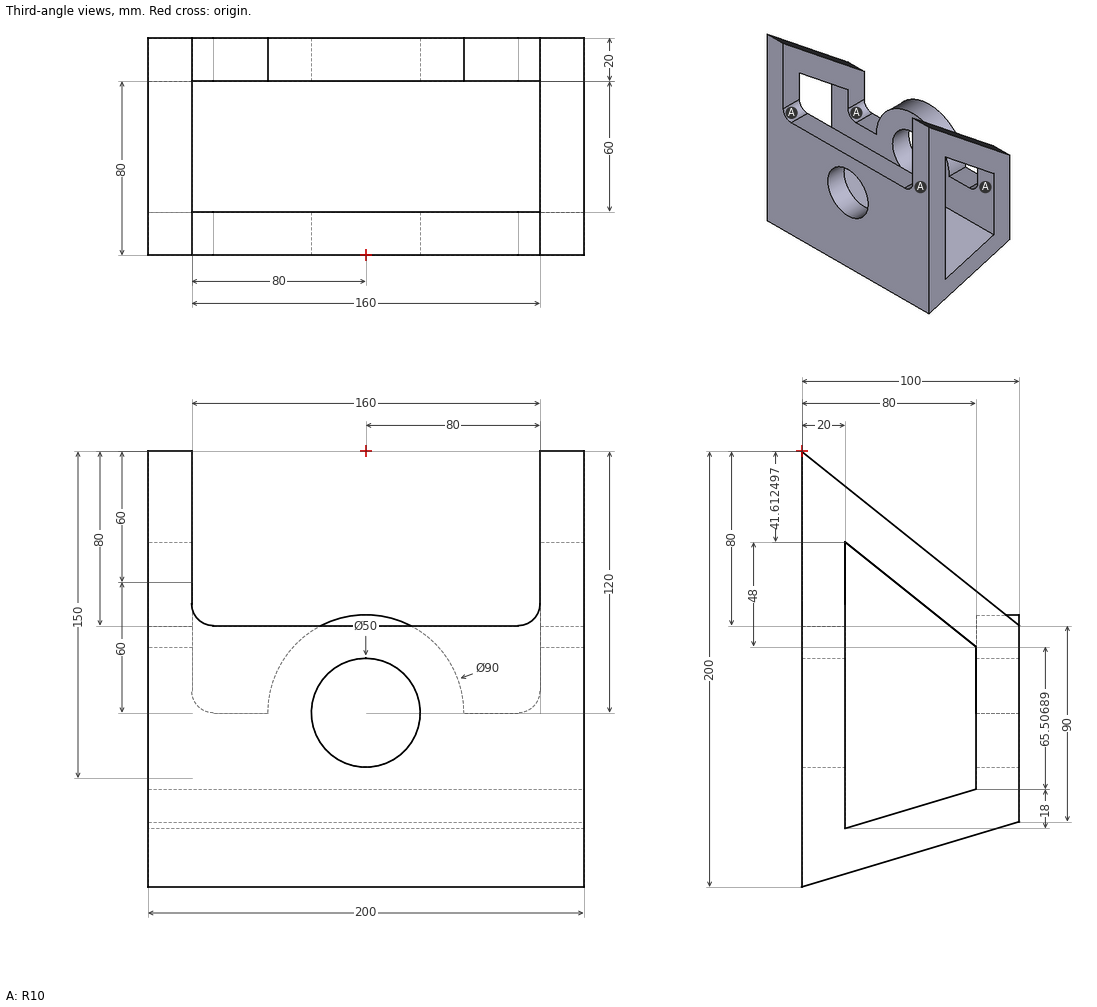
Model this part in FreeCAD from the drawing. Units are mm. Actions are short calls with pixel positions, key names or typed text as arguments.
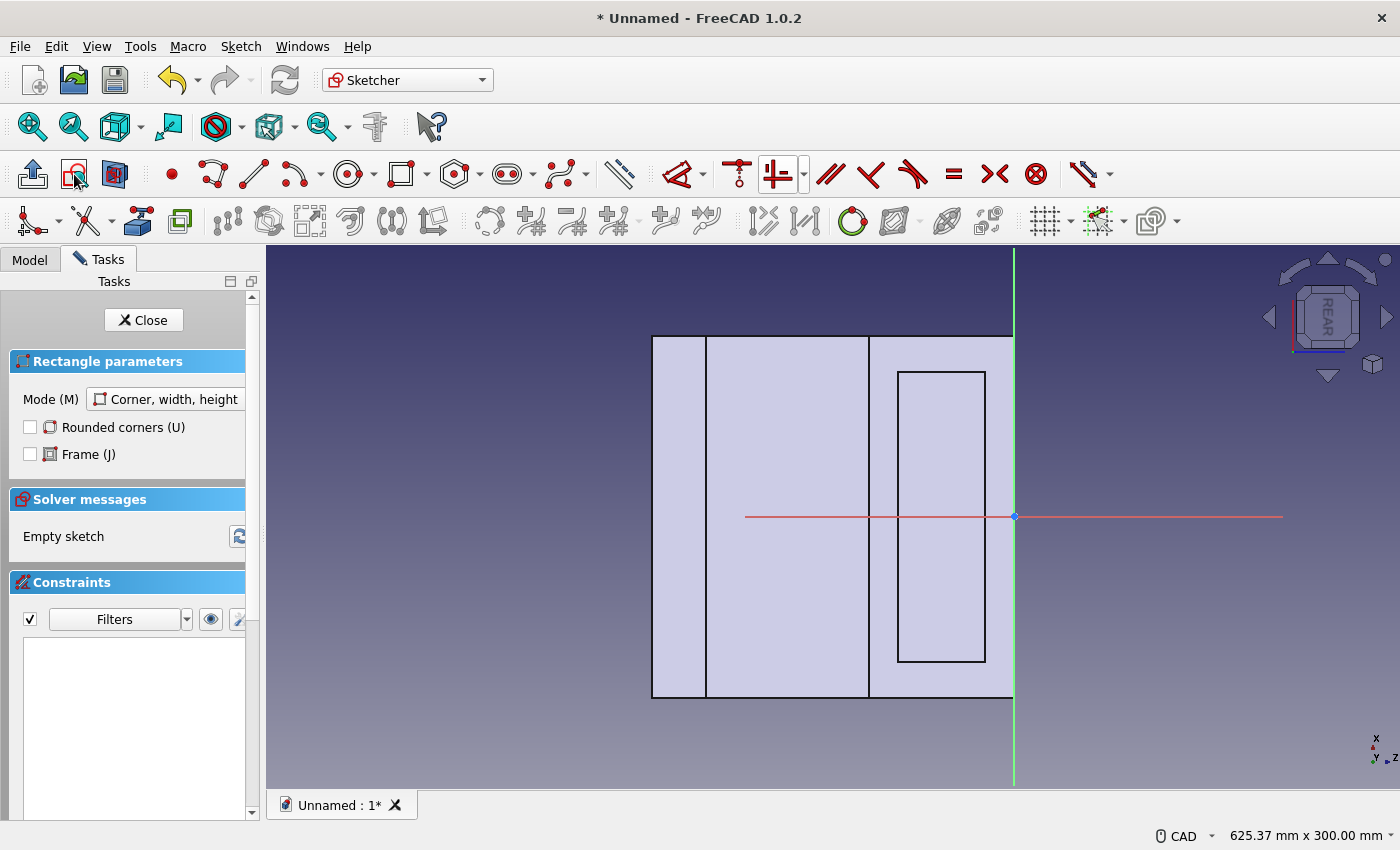
click(797, 372)
move(906, 662)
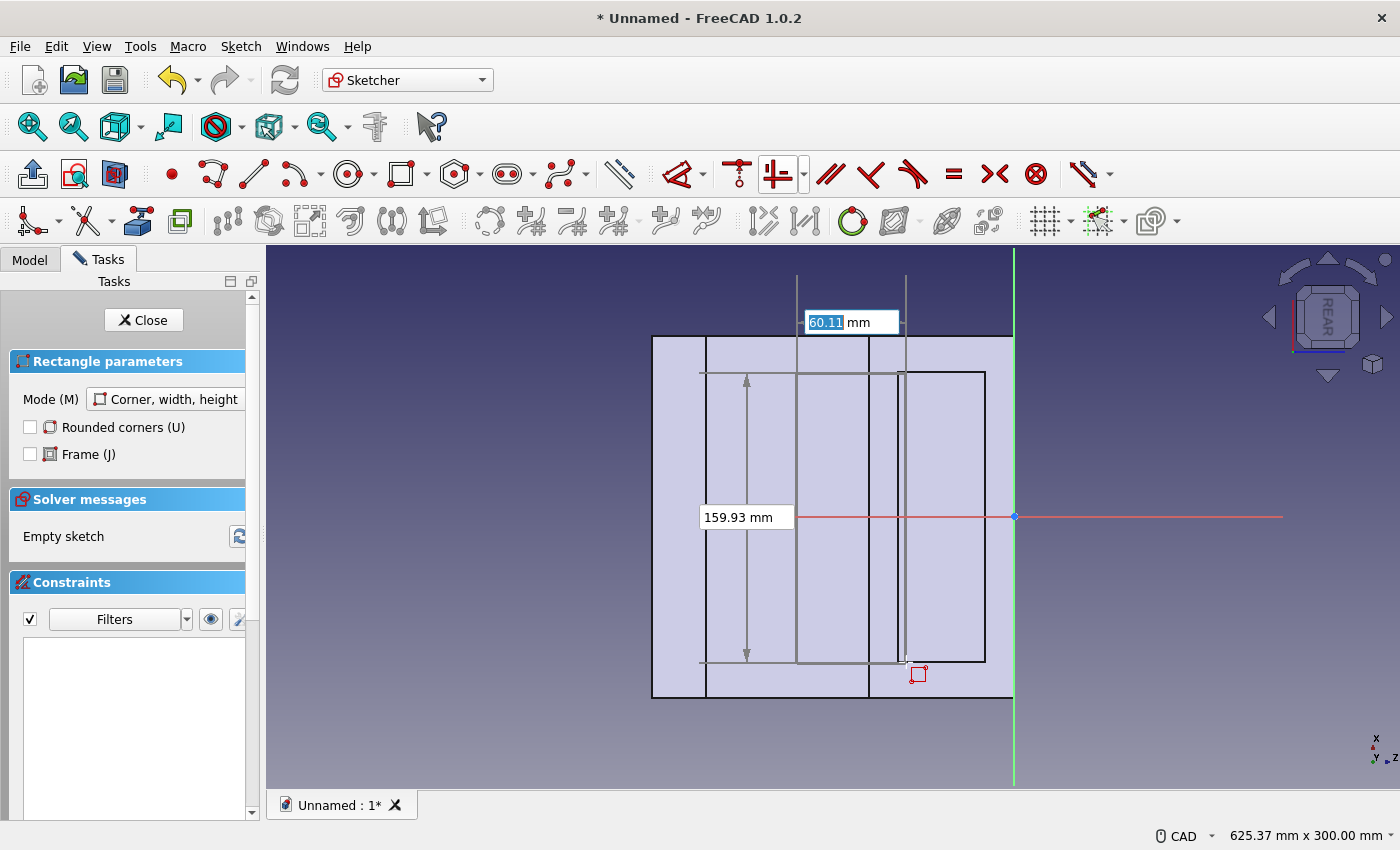
text(60)
key(Tab)
text(160)
key(Return)
key(Escape)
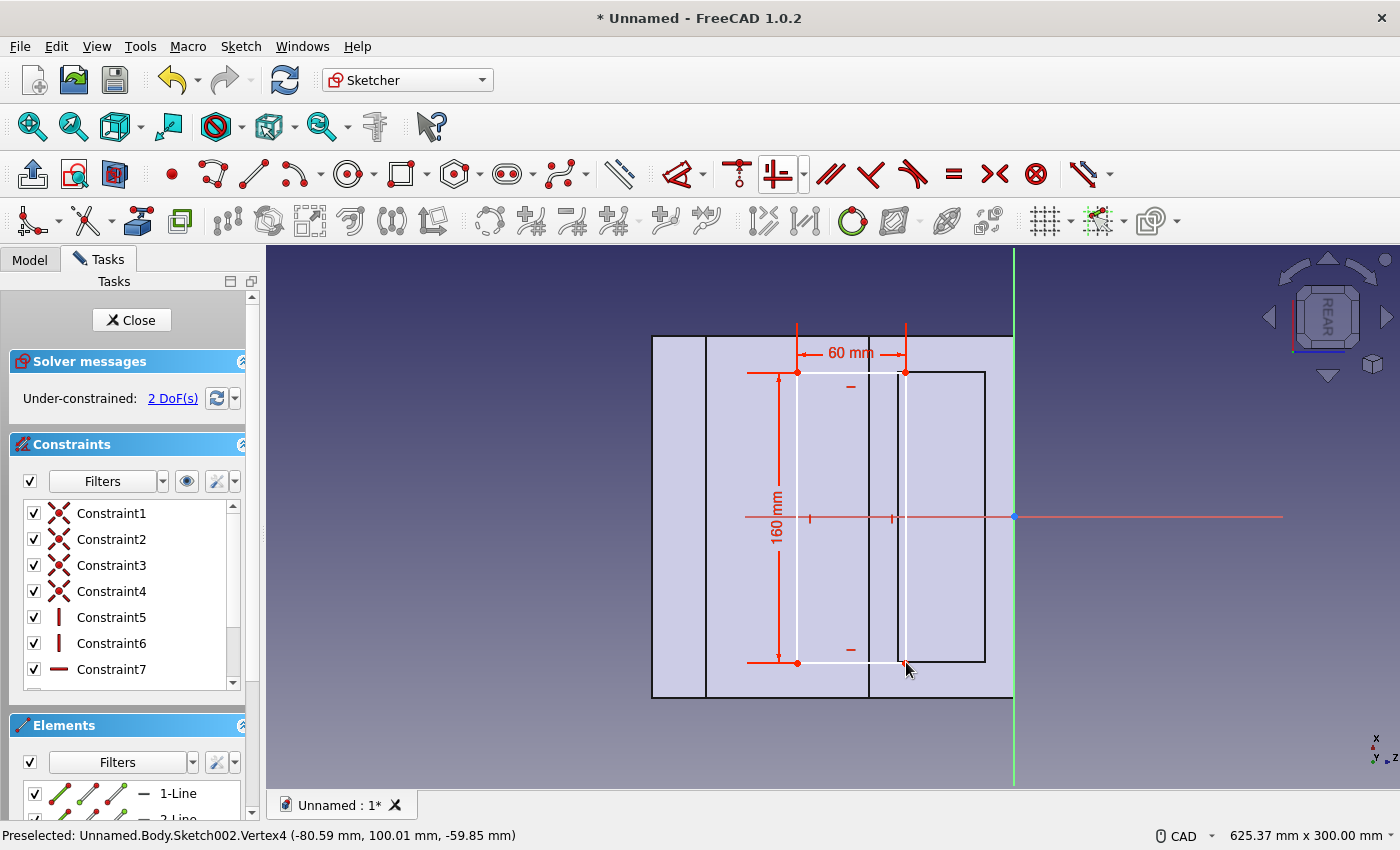
key(d)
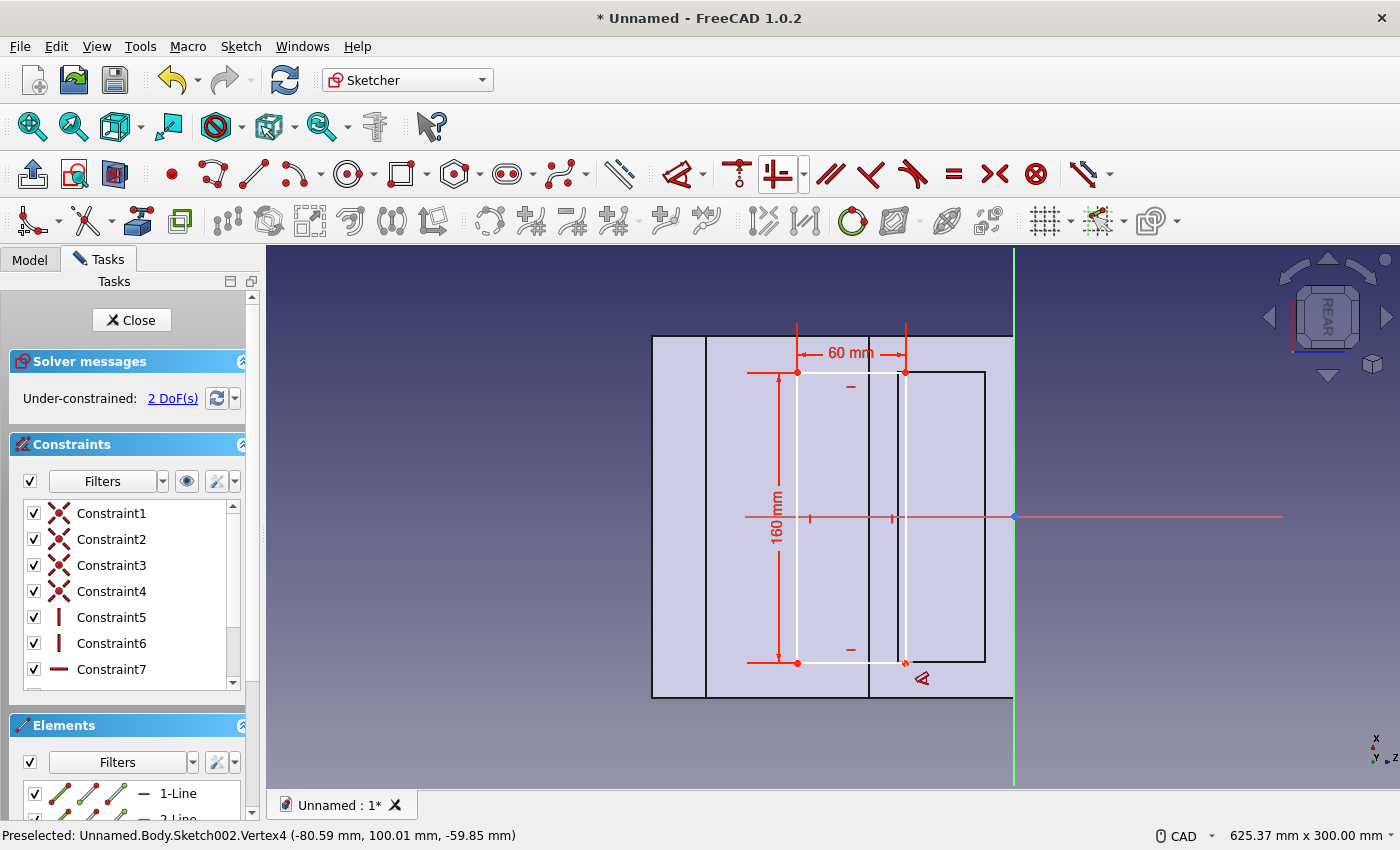
click(797, 373)
click(1048, 445)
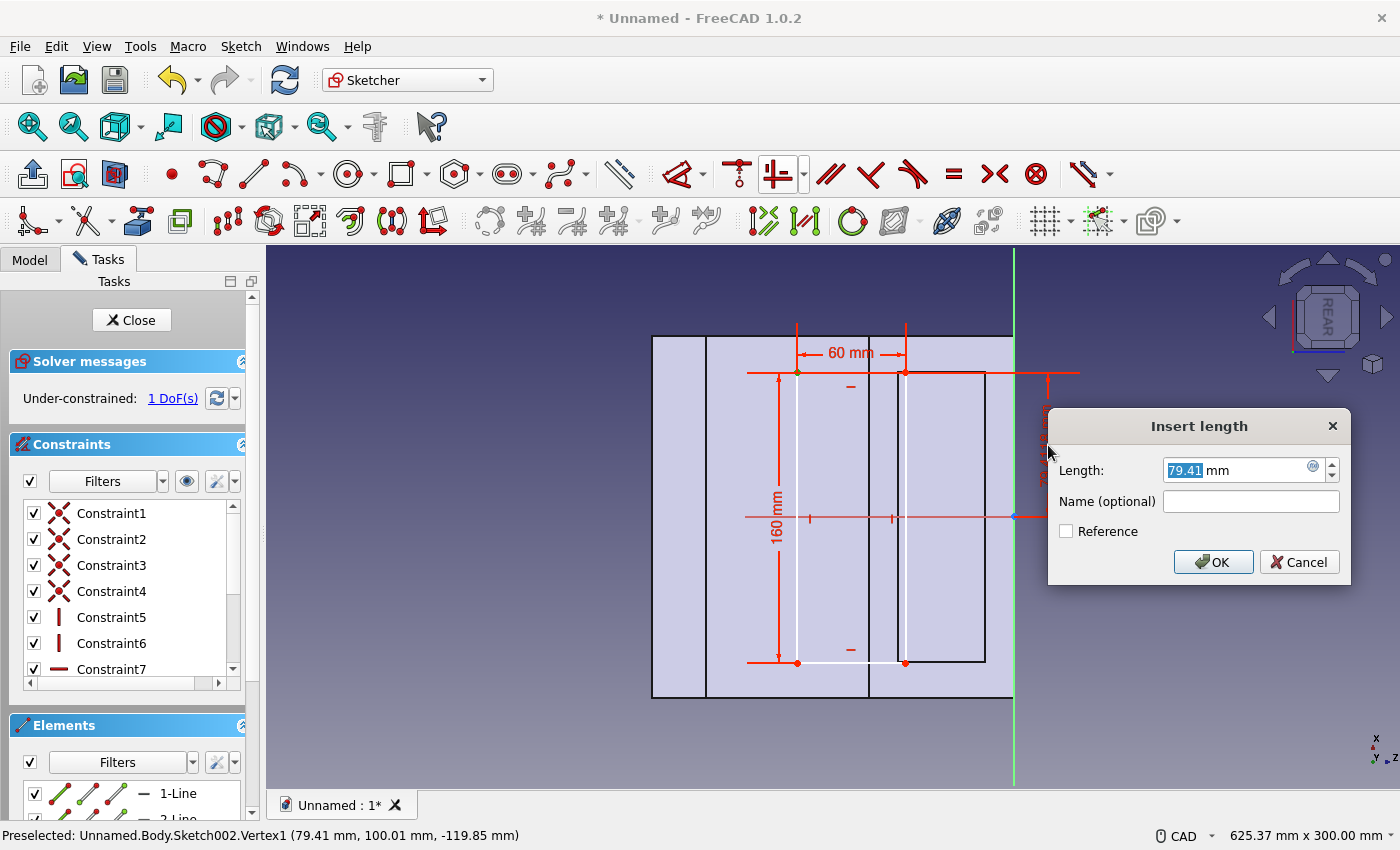
text(80)
key(Return)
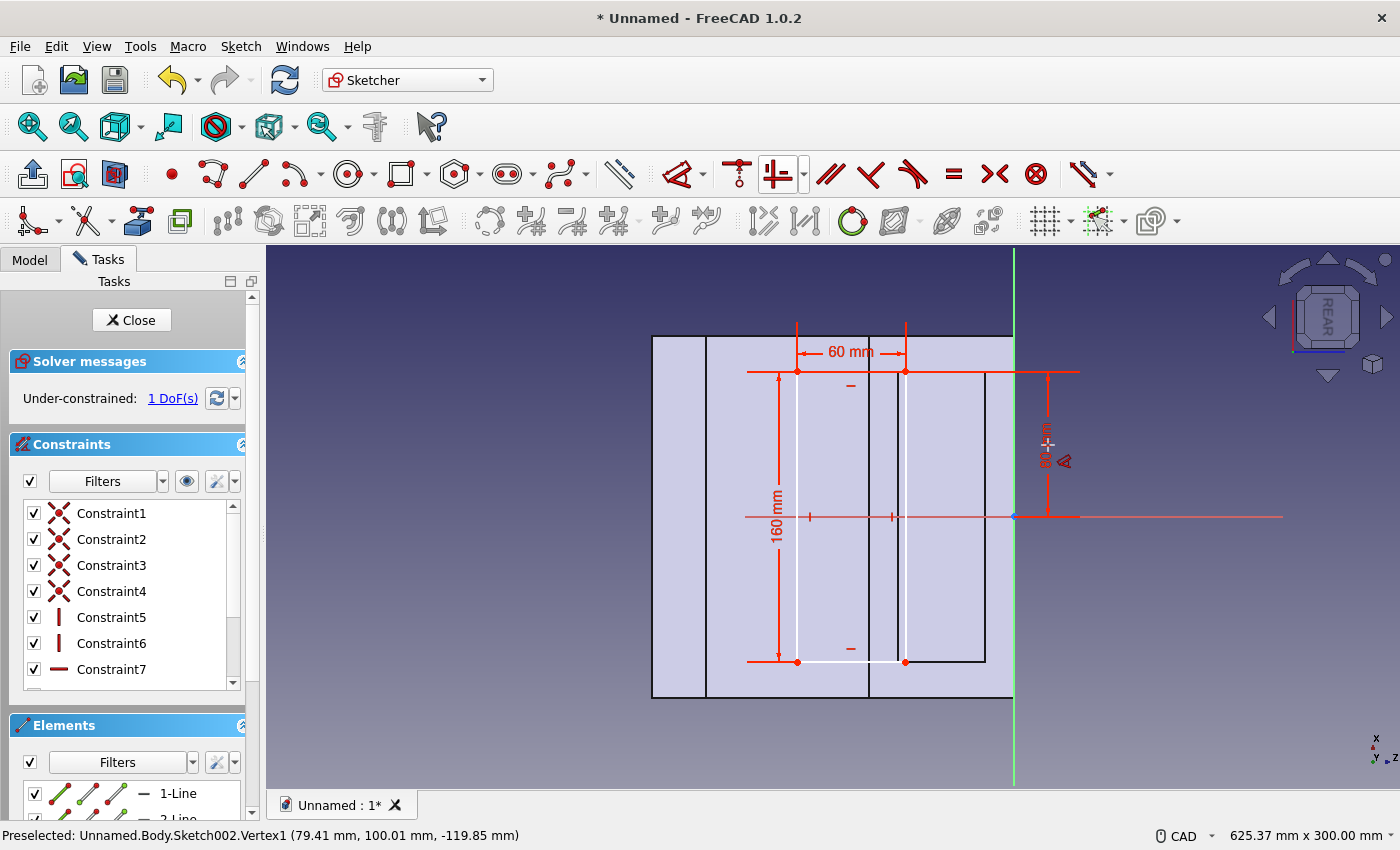
click(906, 662)
click(960, 696)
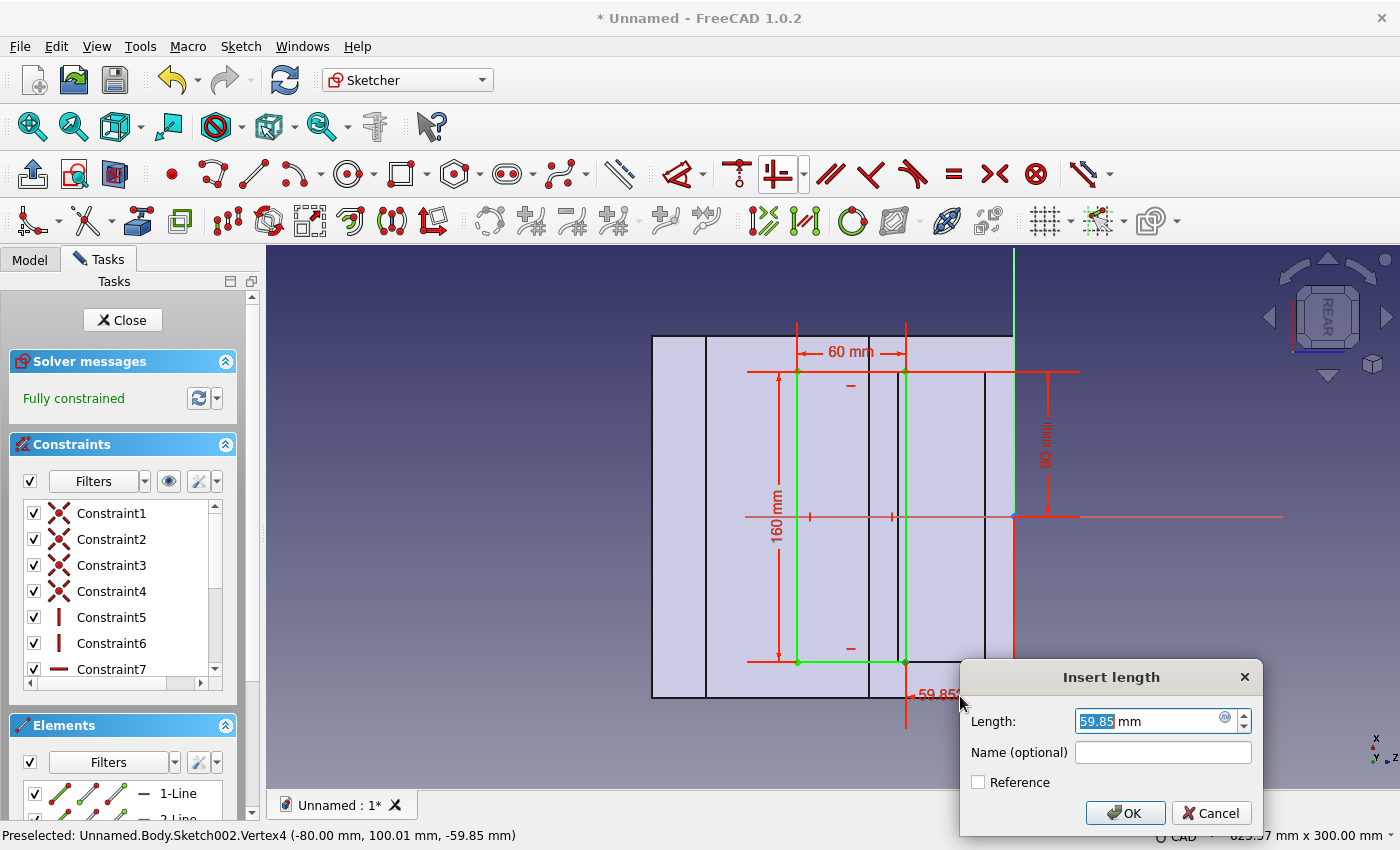
text(60)
key(Return)
key(Escape)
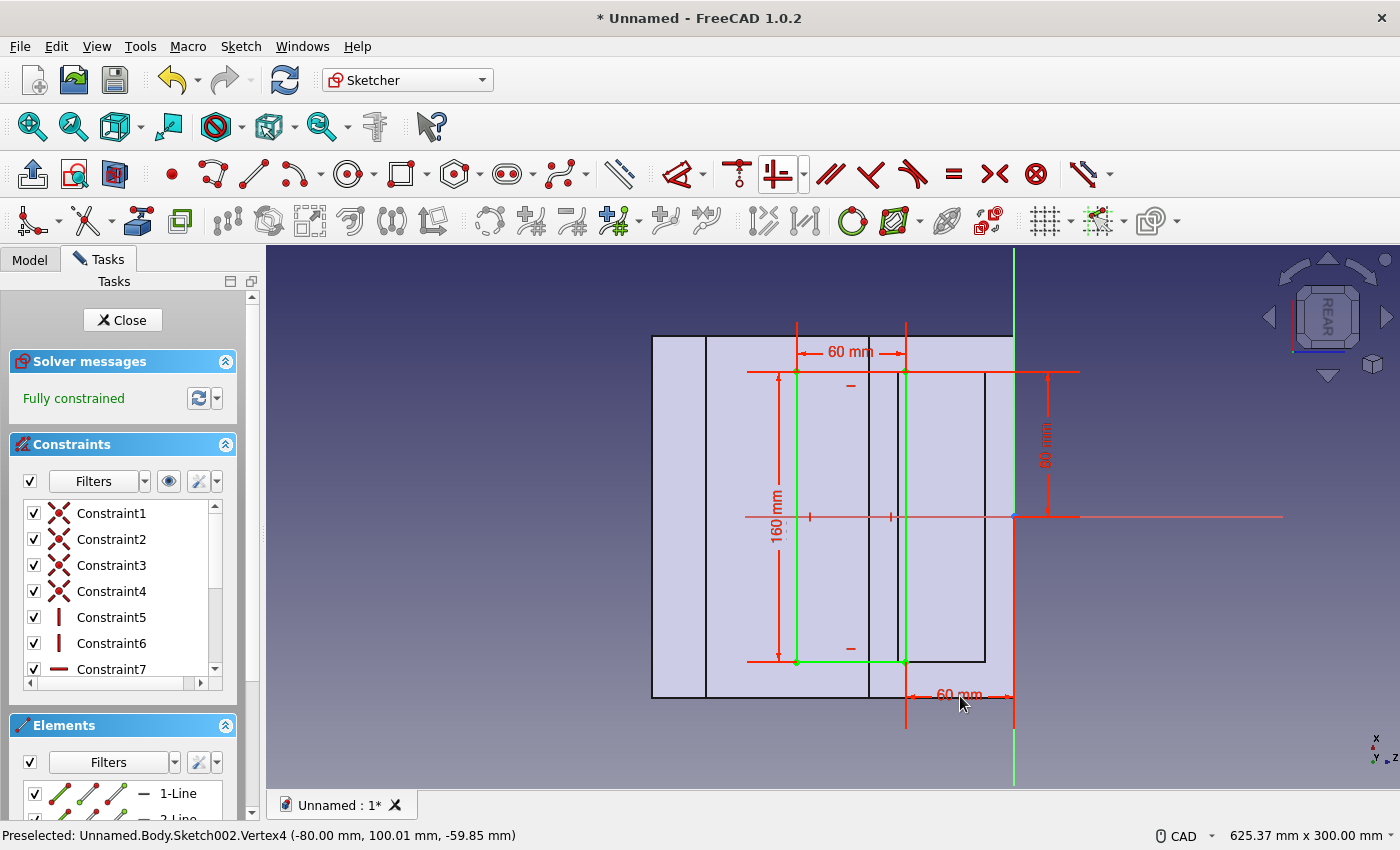
click(123, 320)